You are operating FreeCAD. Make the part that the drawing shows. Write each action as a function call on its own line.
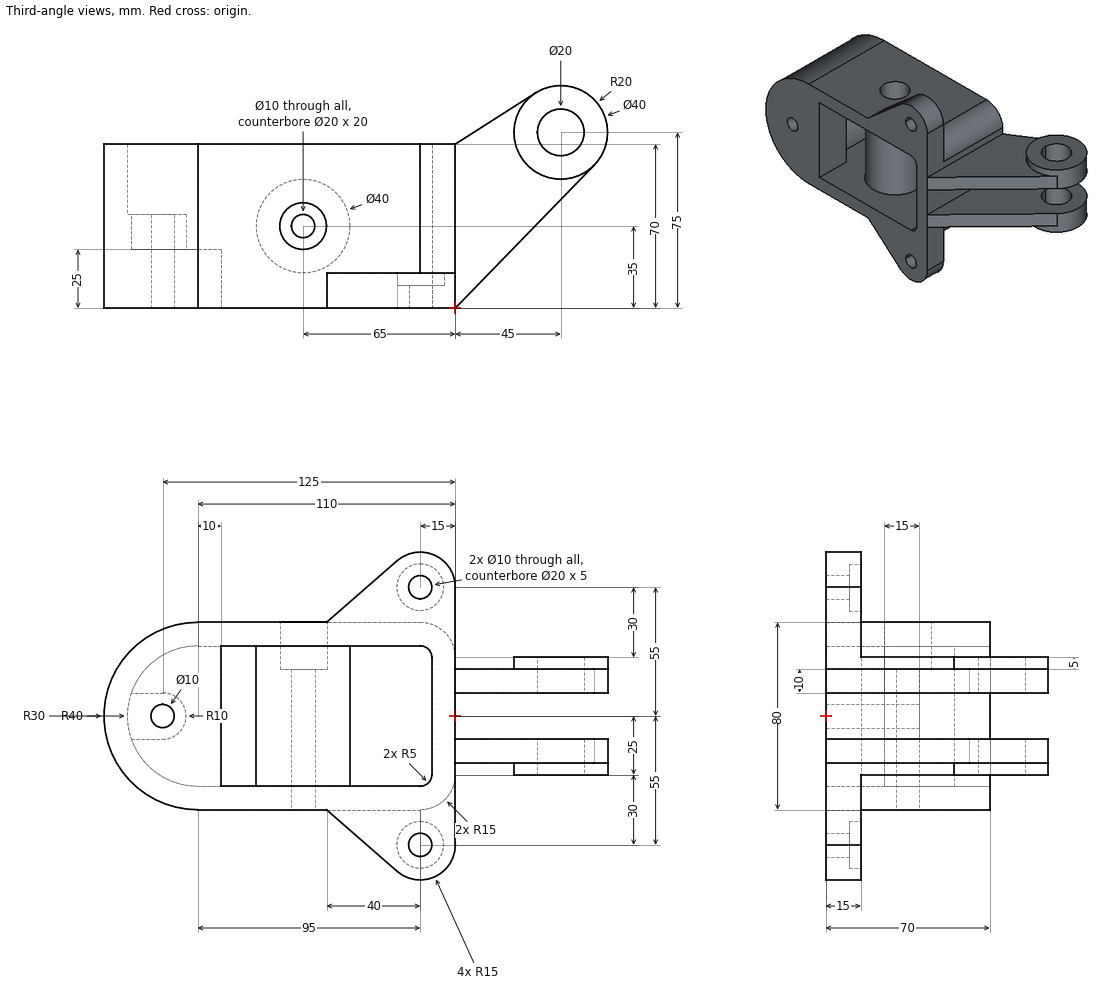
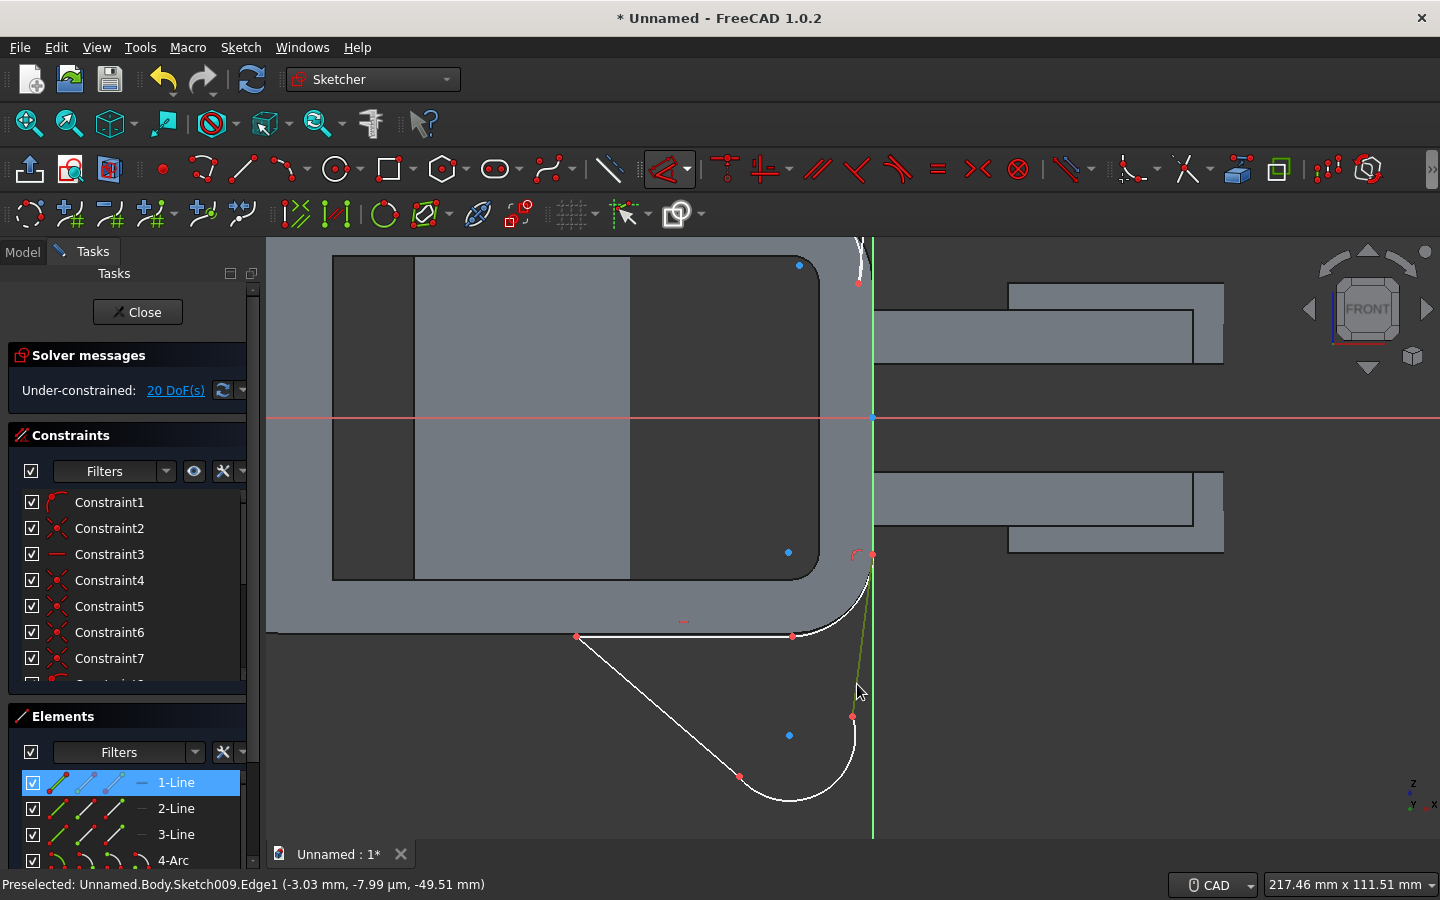
click(786, 801)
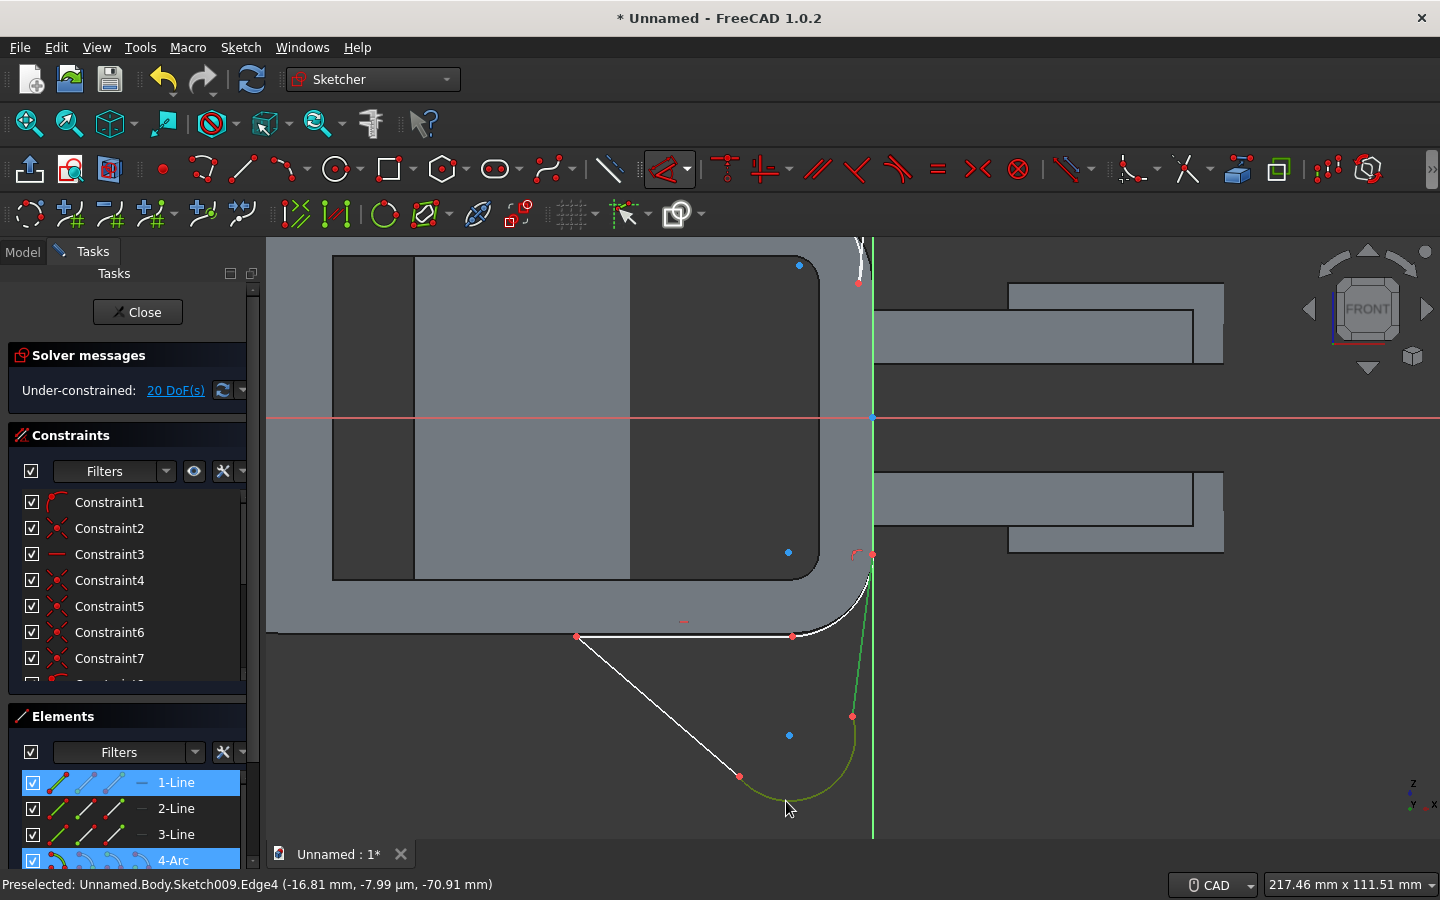
key(t)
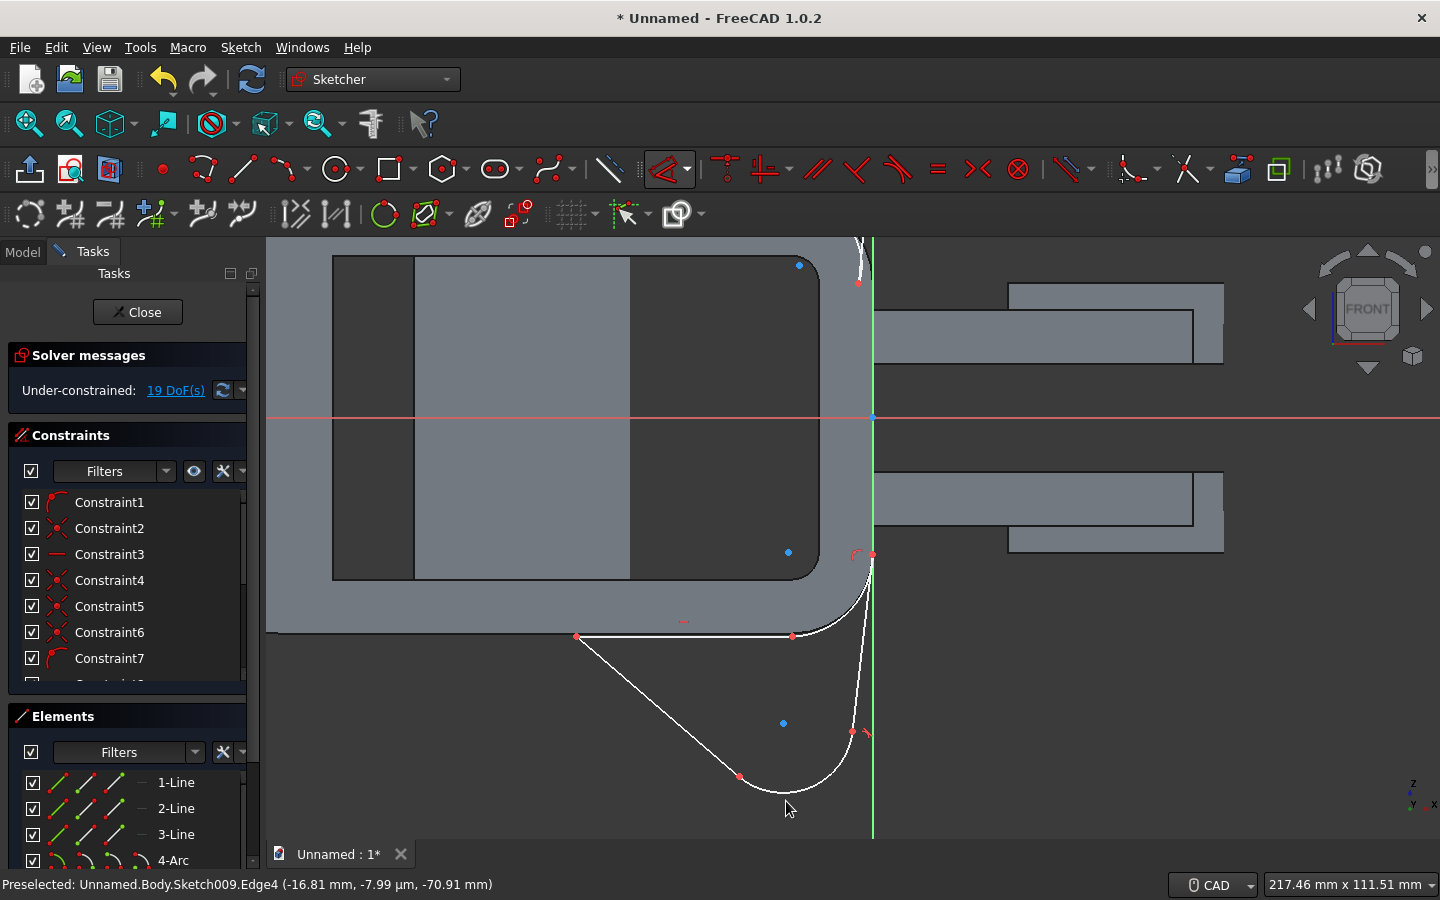
click(859, 678)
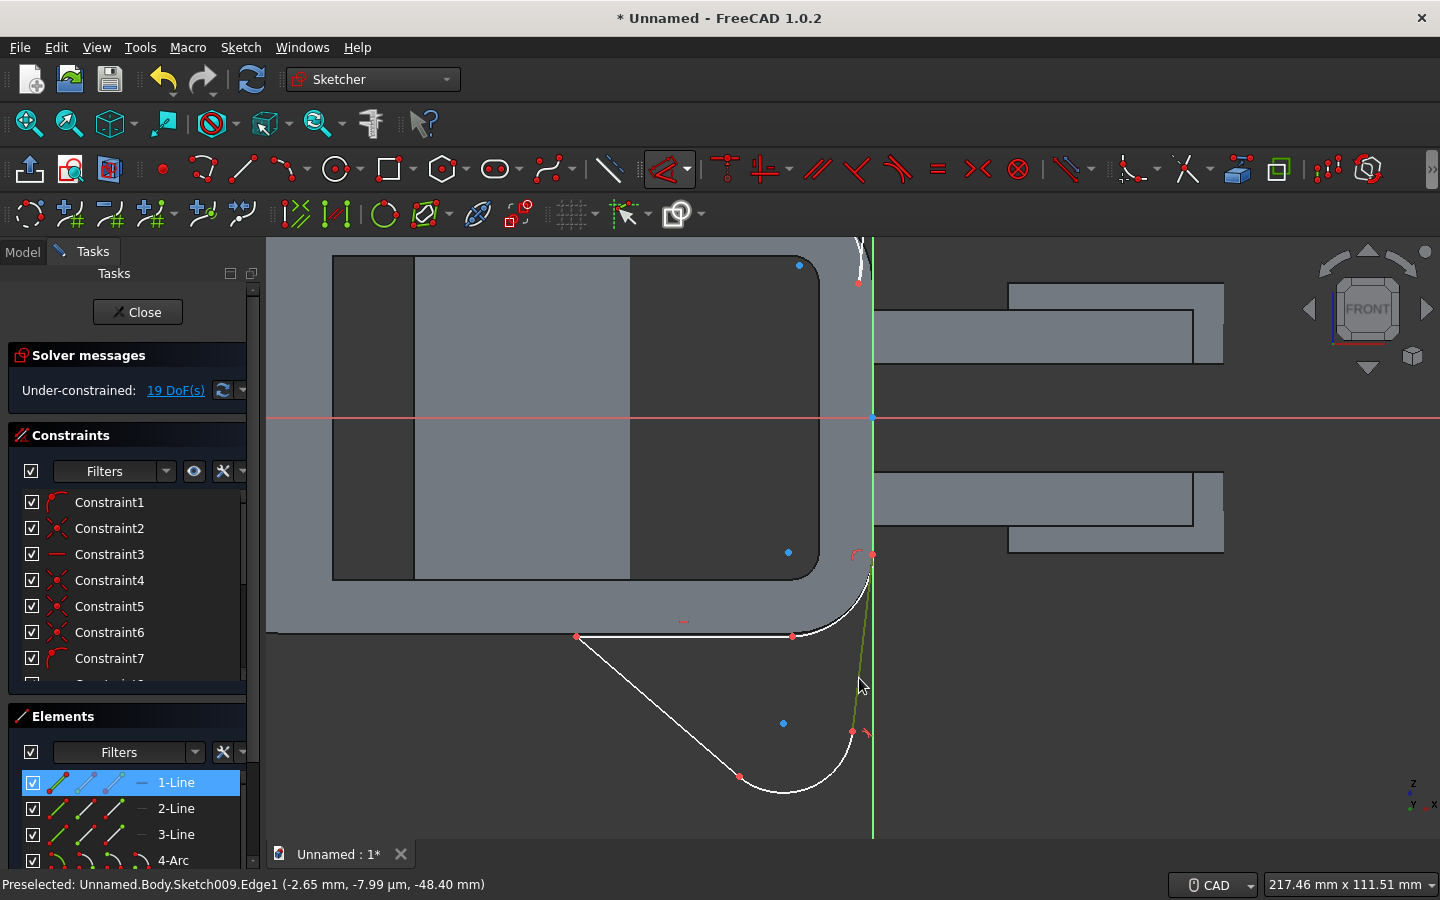
click(829, 627)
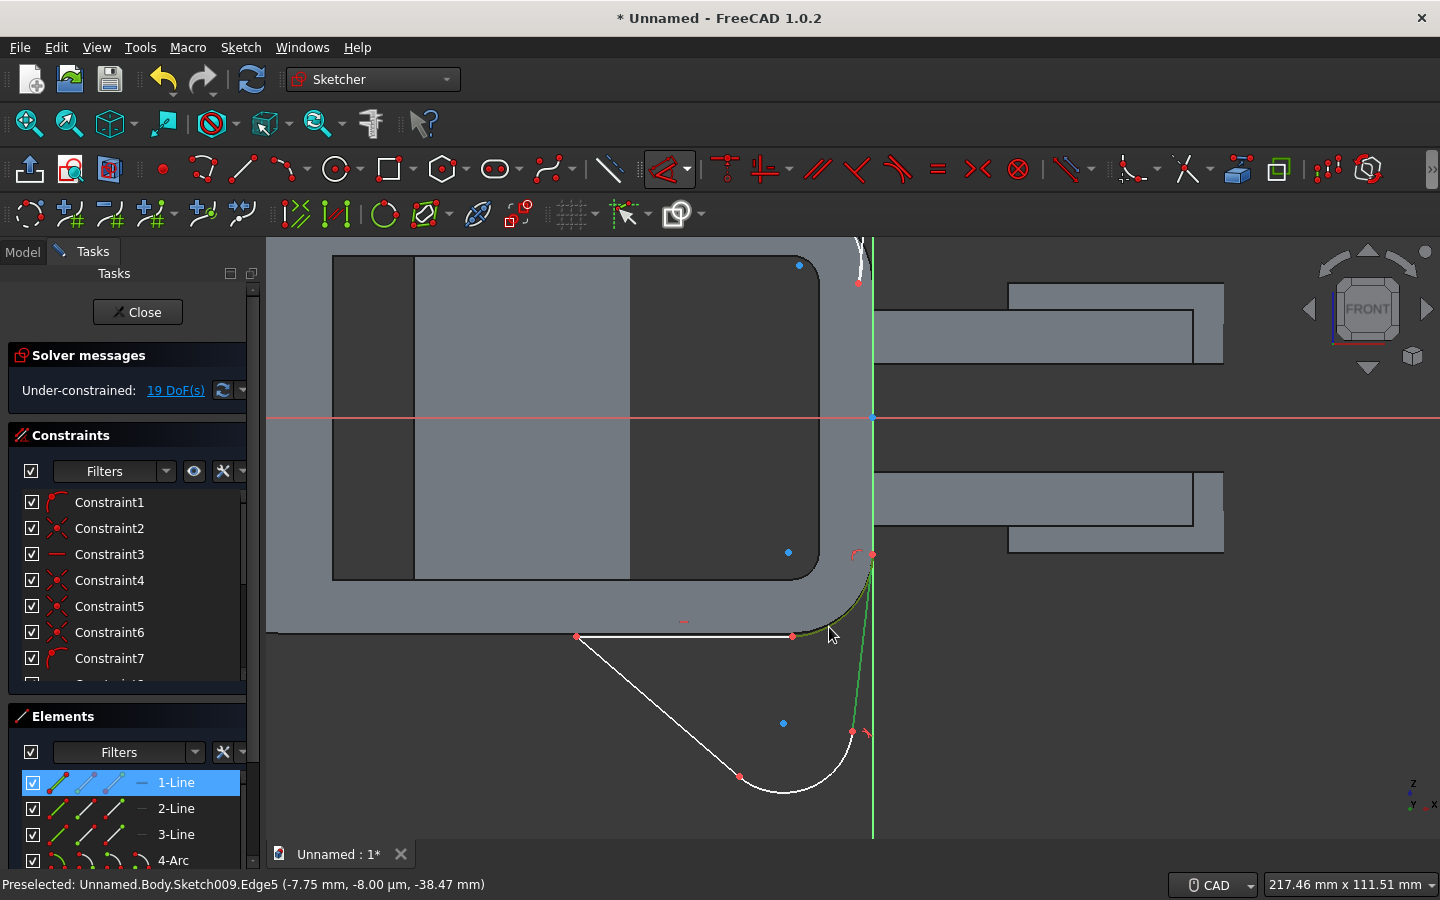
key(t)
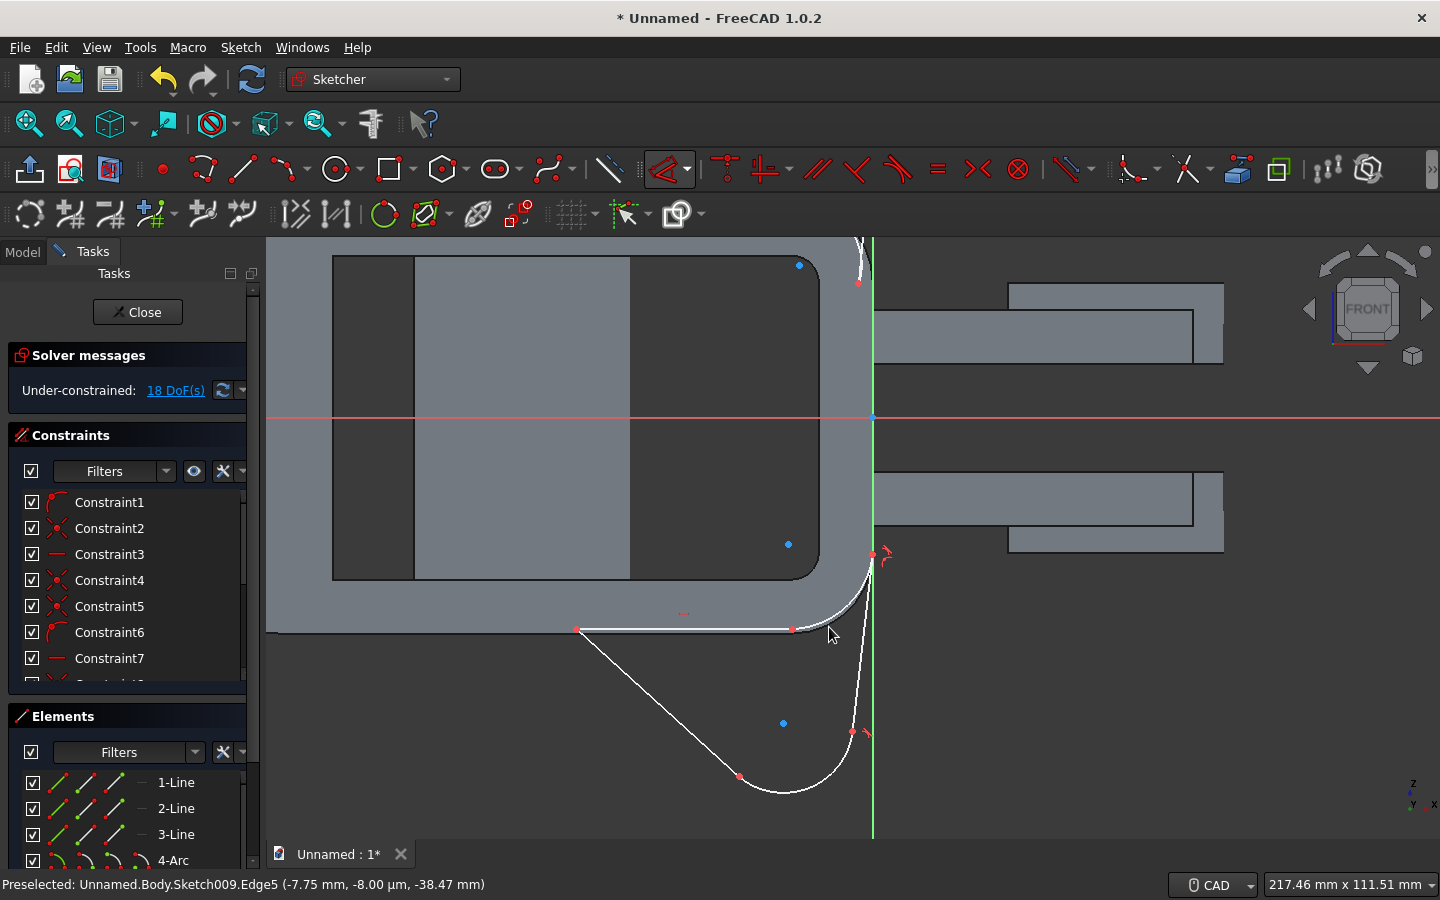
click(690, 732)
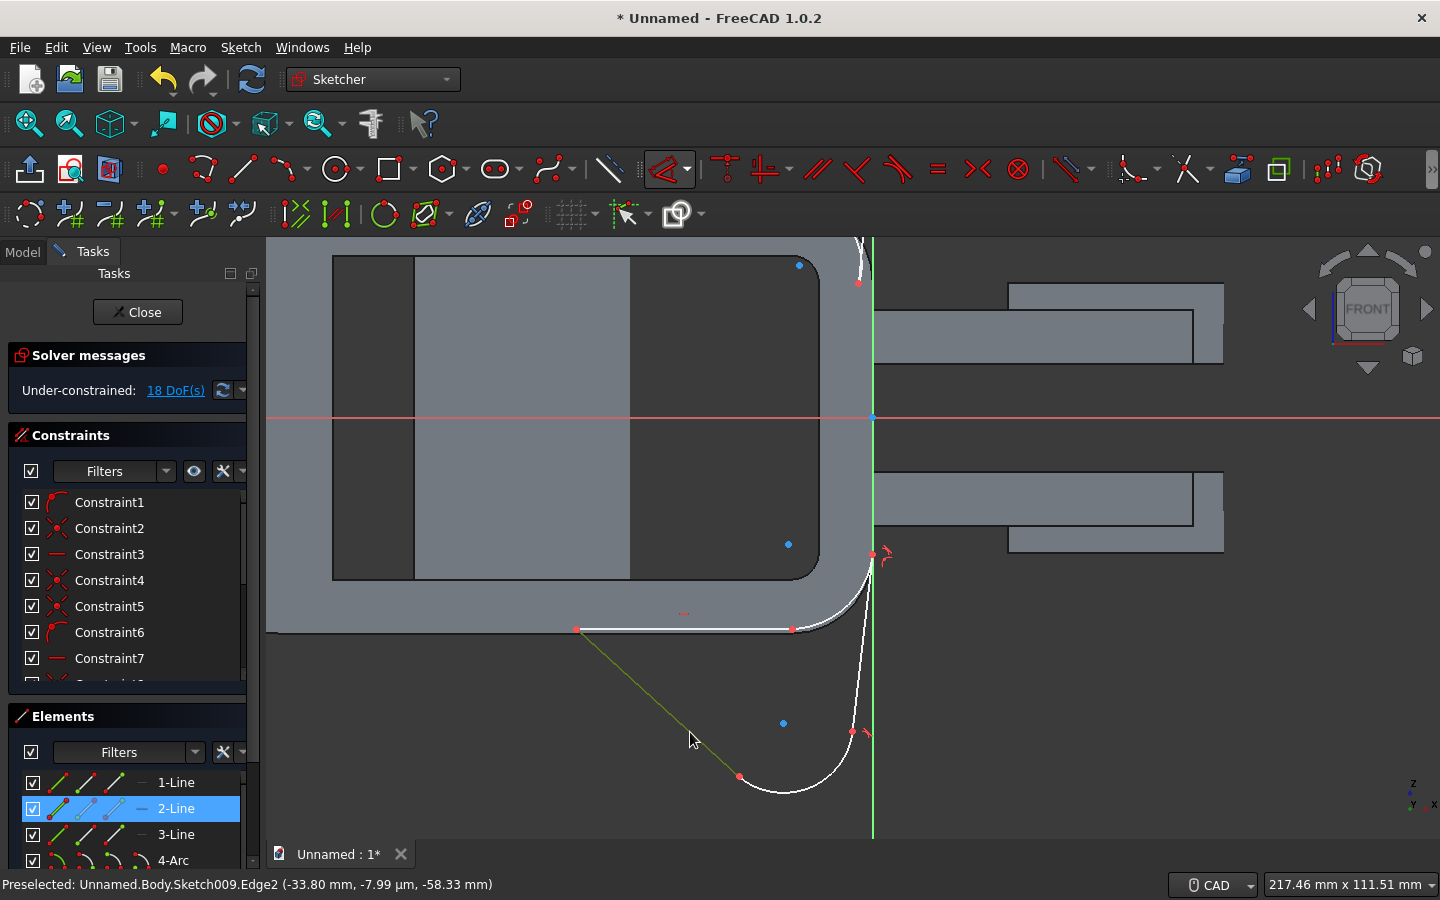
click(780, 793)